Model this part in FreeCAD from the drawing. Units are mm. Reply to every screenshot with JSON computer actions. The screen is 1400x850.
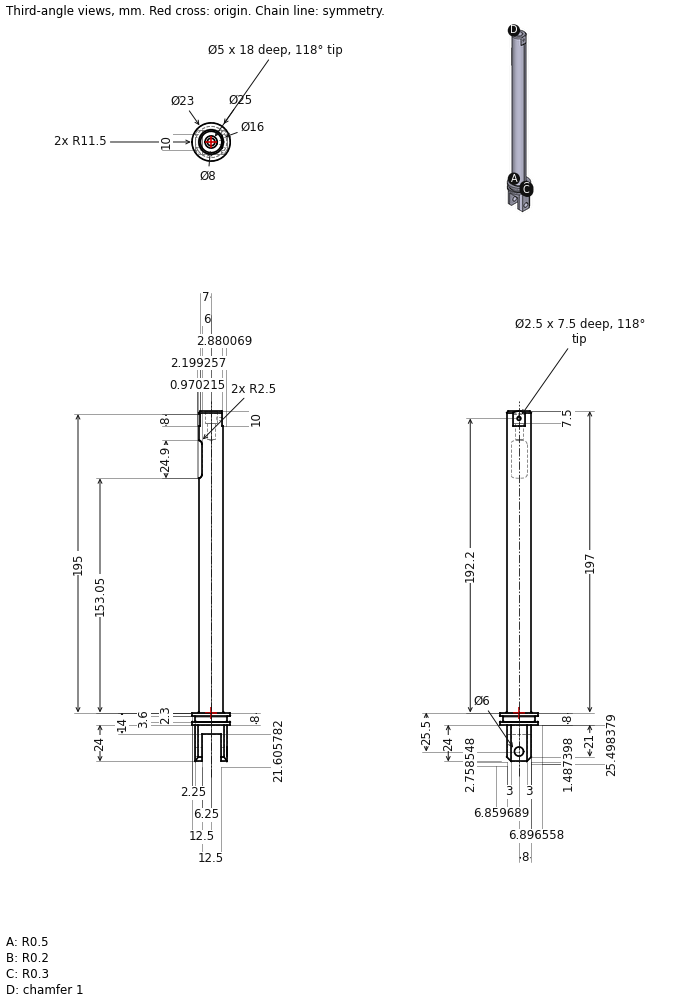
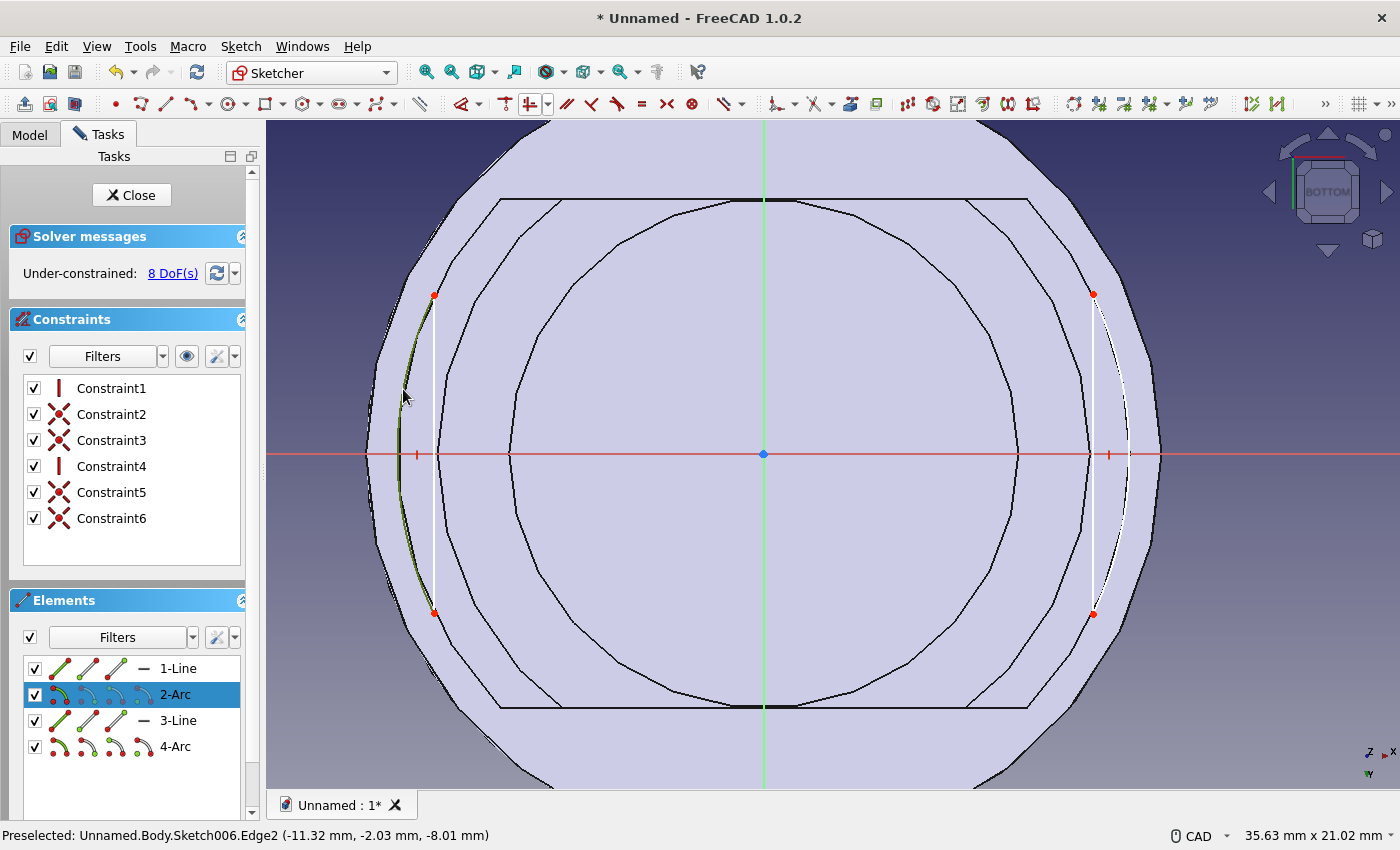
{"action": "left_click", "coordinate": [1124, 520]}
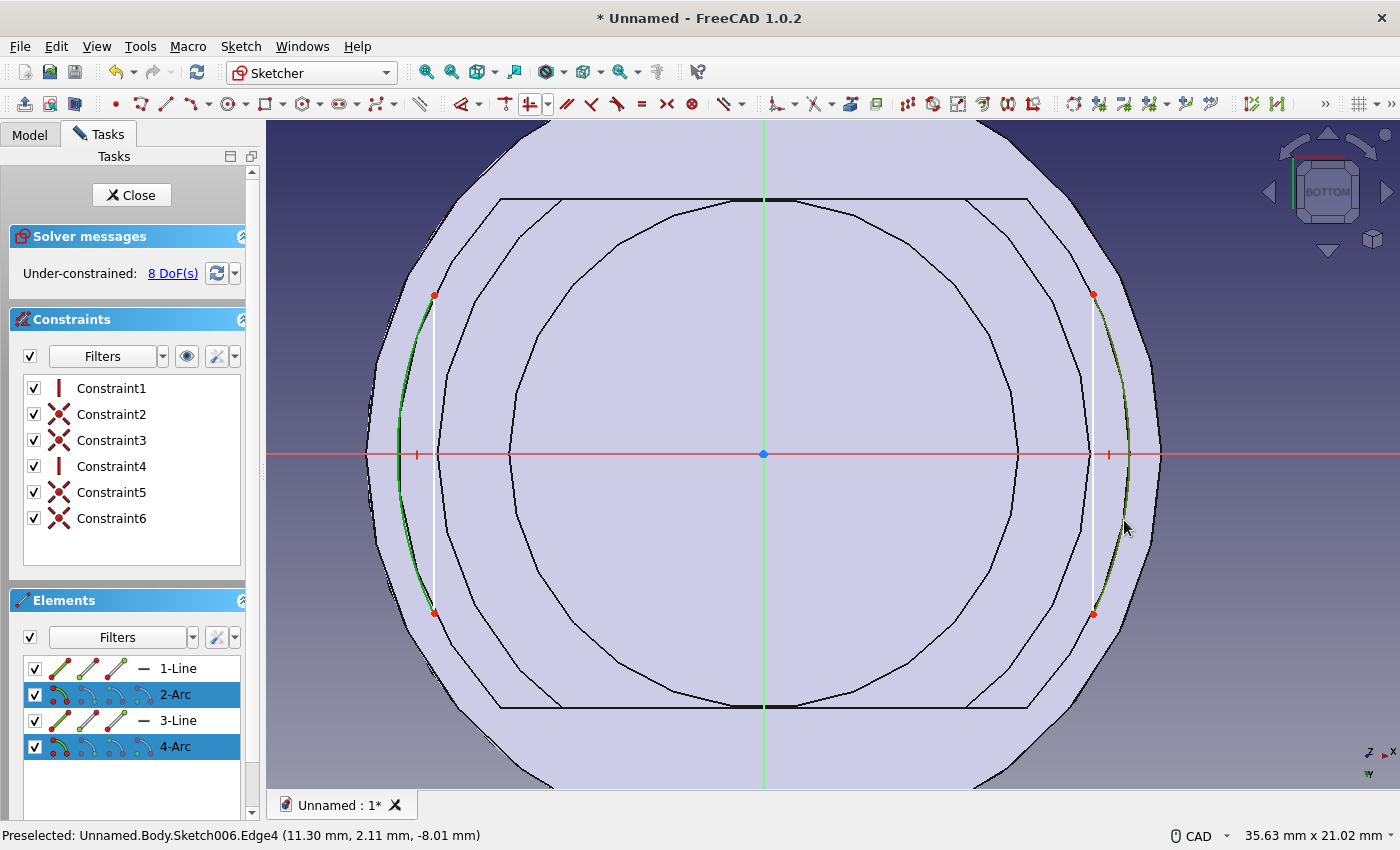
{"action": "left_click", "coordinate": [505, 104]}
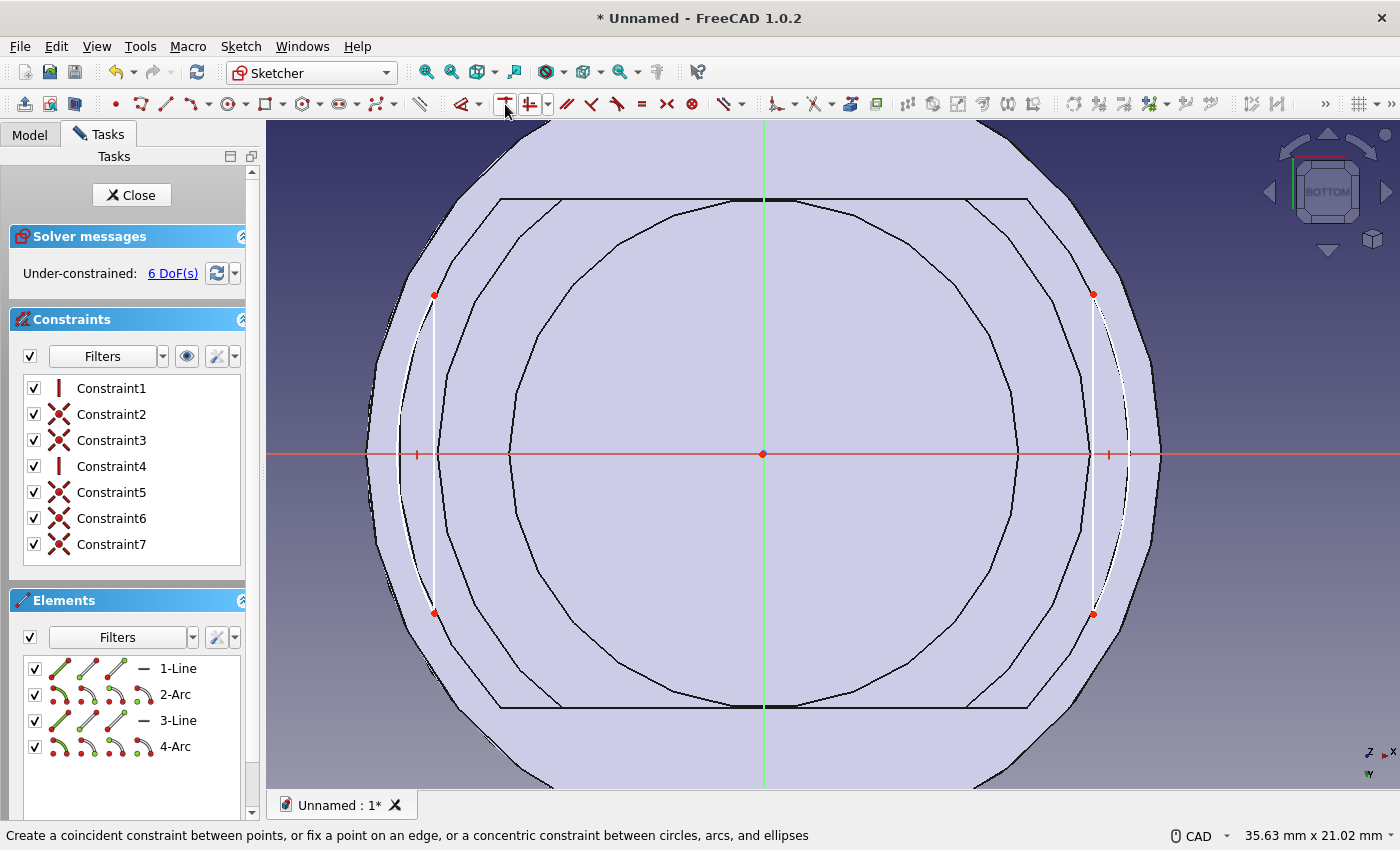
{"action": "left_click_drag", "start_coordinate": [752, 444], "coordinate": [774, 465]}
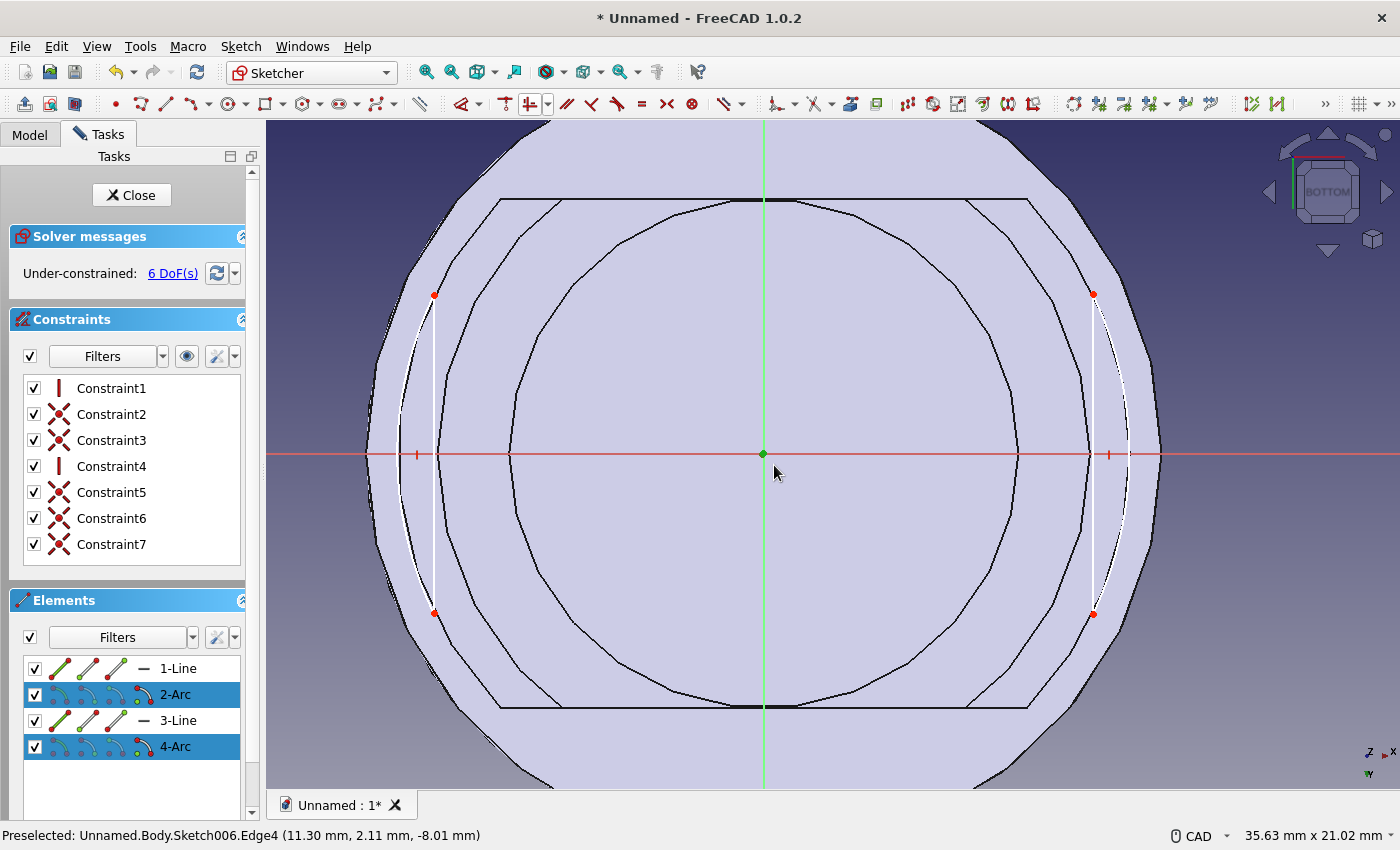
{"action": "left_click", "coordinate": [505, 104]}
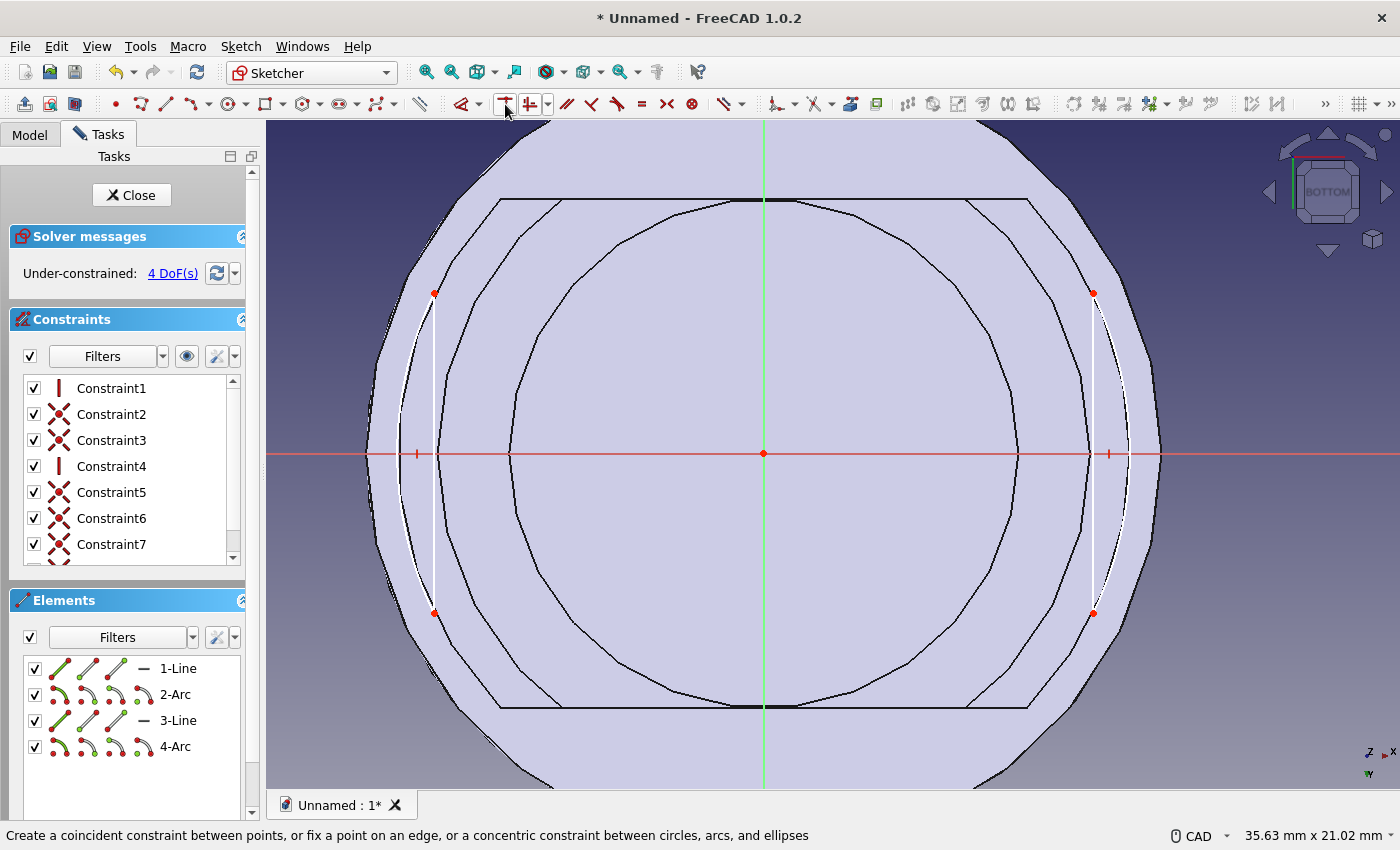
{"action": "left_click", "coordinate": [403, 388]}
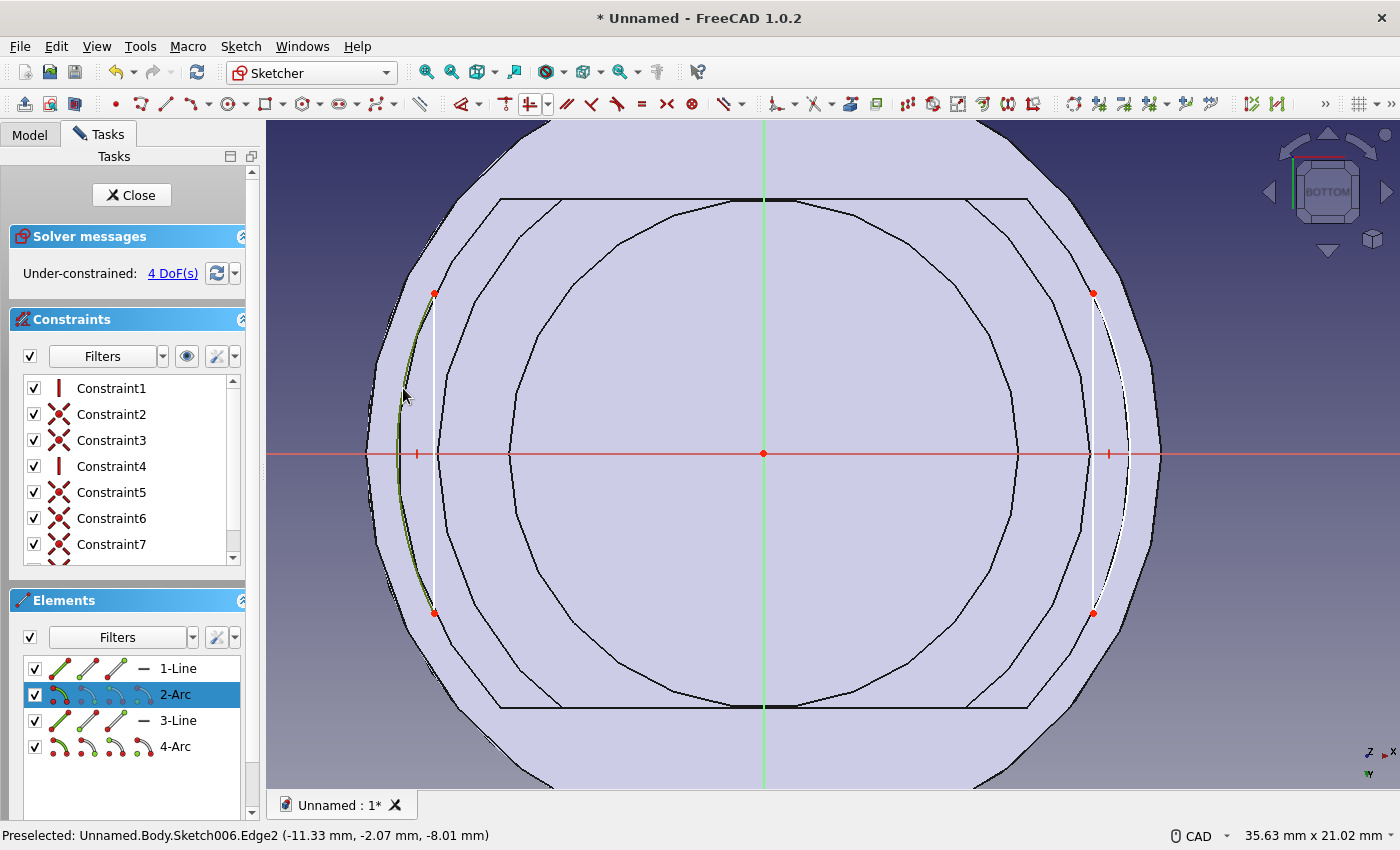
{"action": "left_click", "coordinate": [1124, 520]}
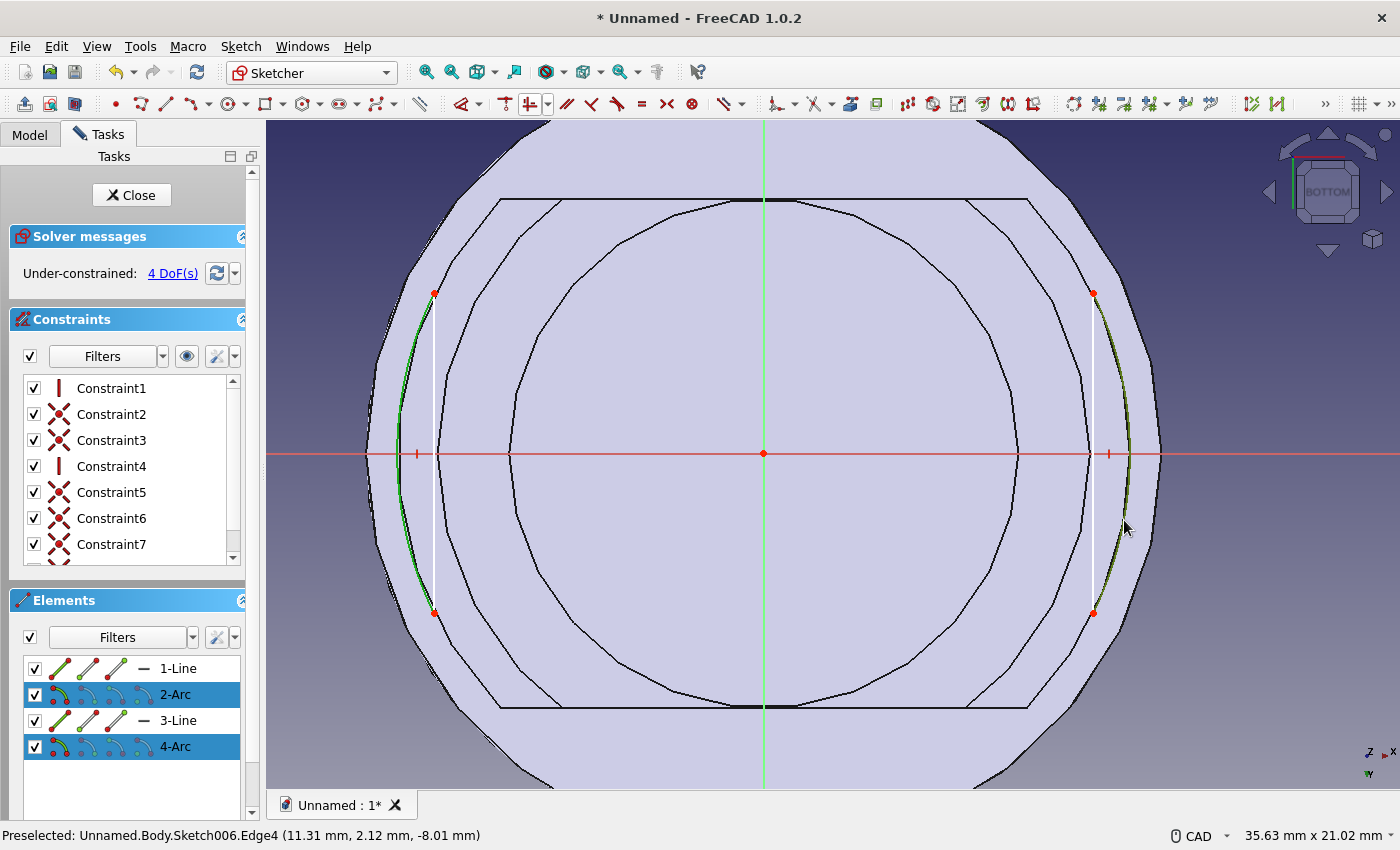
{"action": "left_click", "coordinate": [642, 104]}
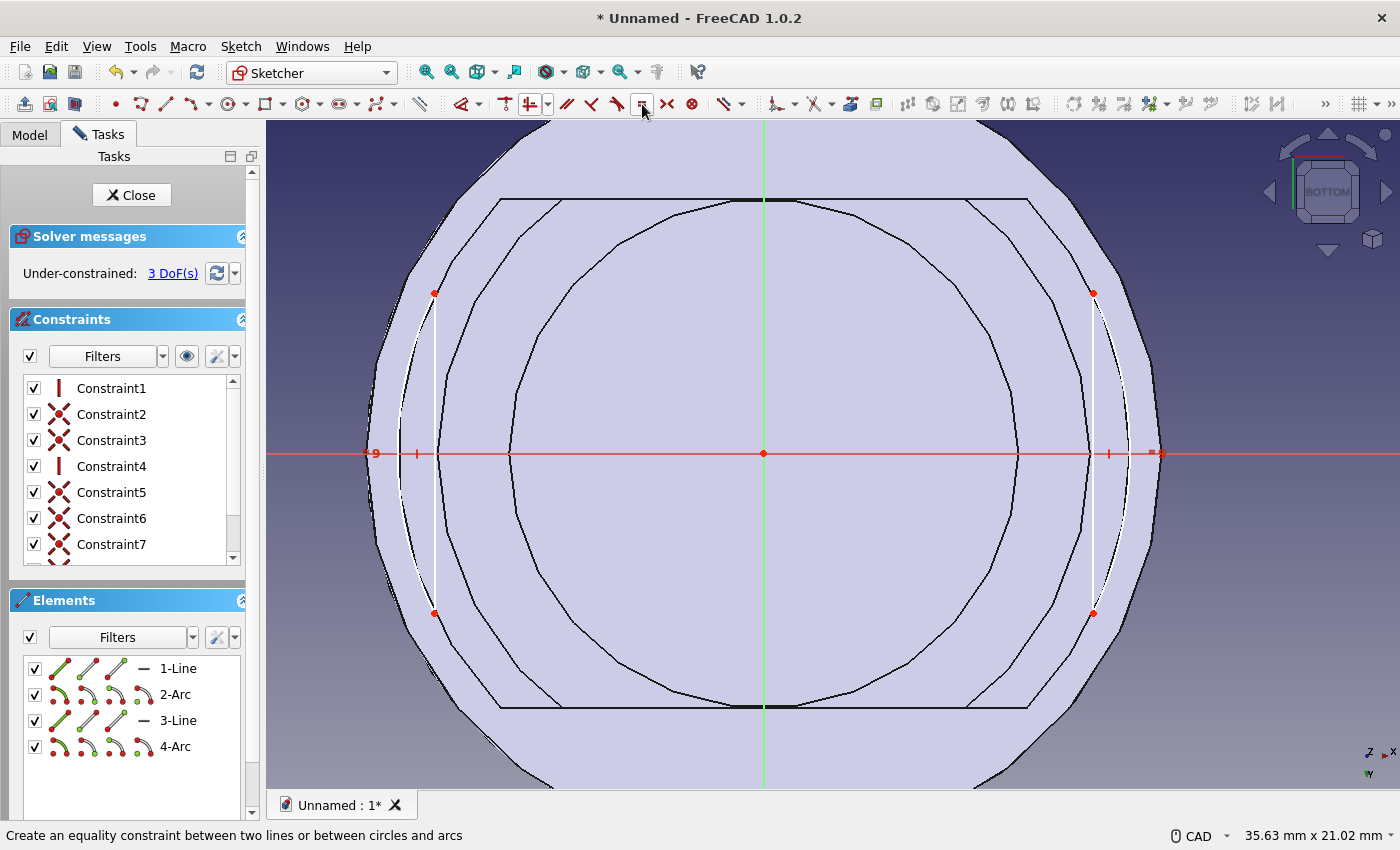
{"action": "left_click", "coordinate": [460, 104]}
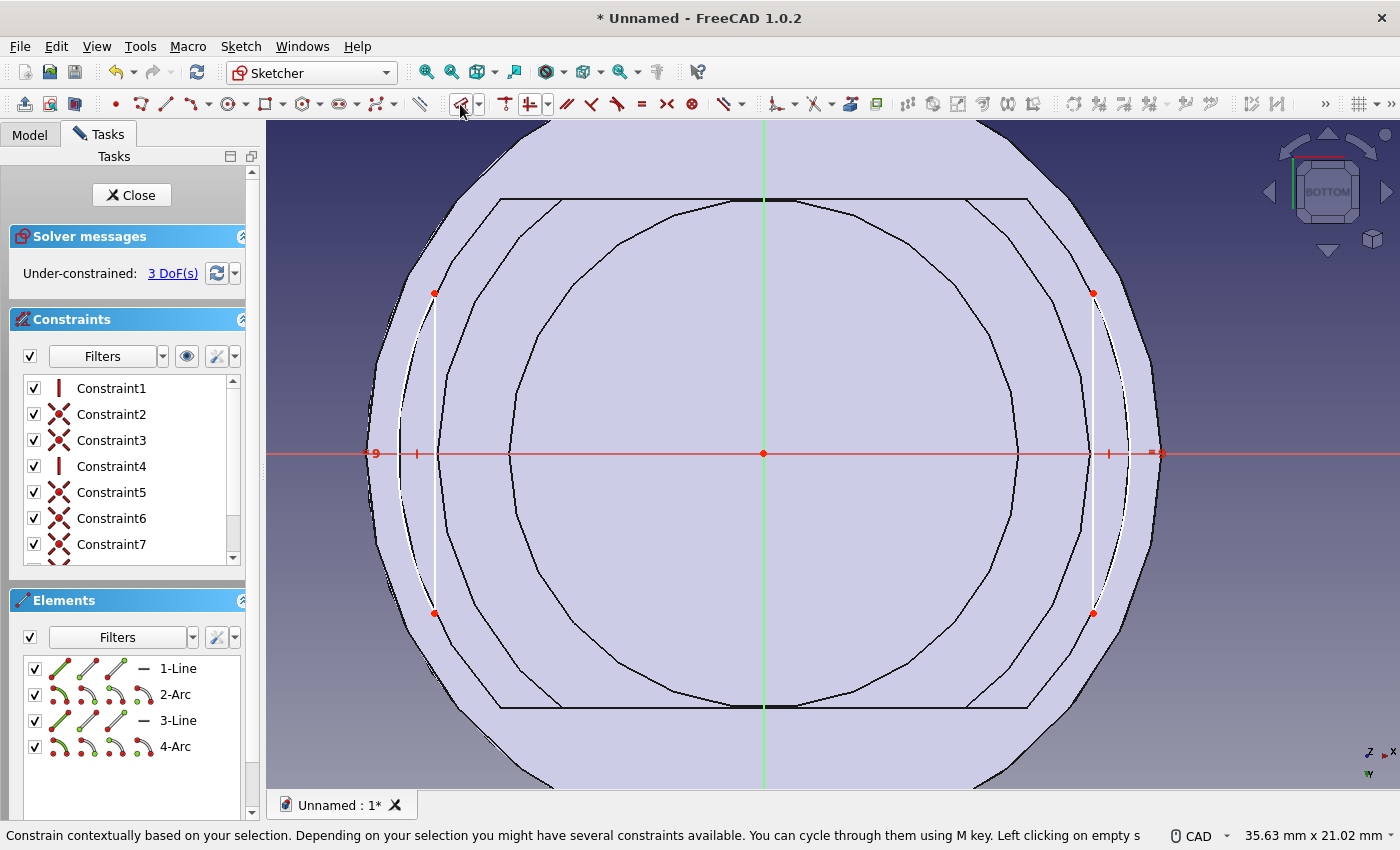
{"action": "left_click", "coordinate": [404, 388]}
{"action": "left_click", "coordinate": [373, 382]}